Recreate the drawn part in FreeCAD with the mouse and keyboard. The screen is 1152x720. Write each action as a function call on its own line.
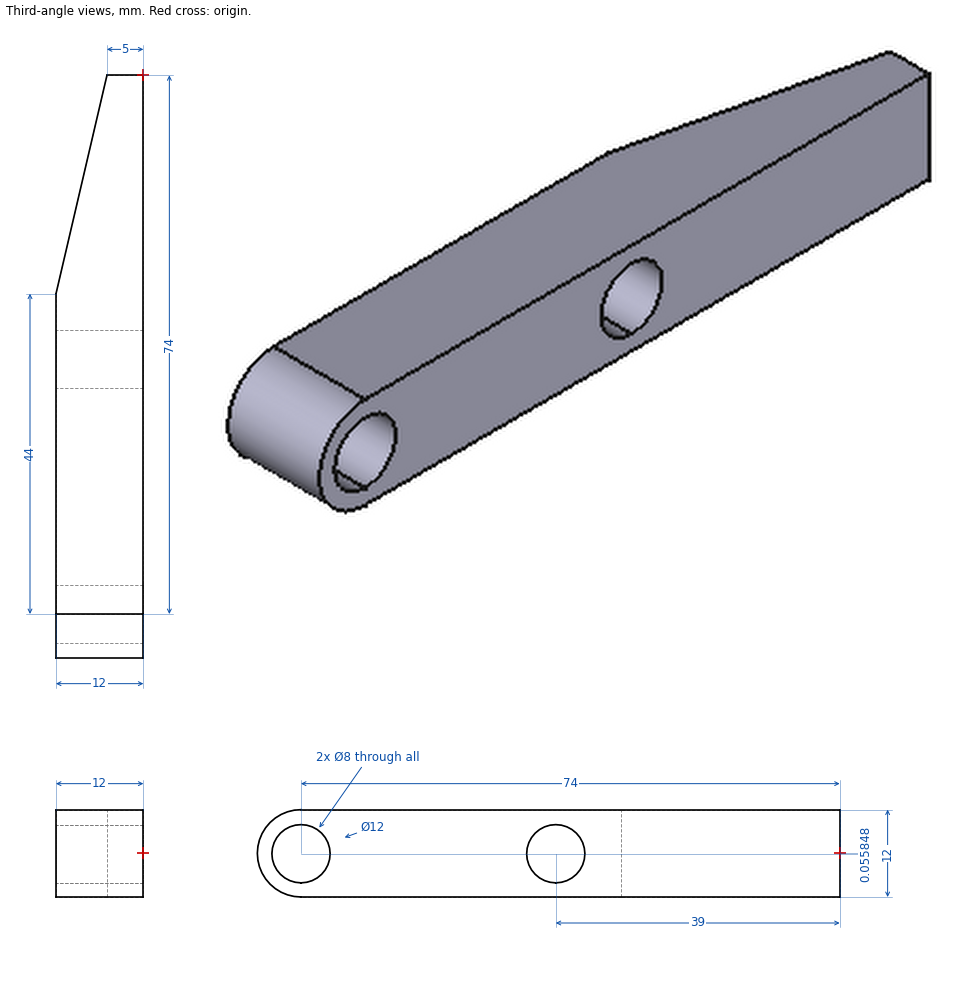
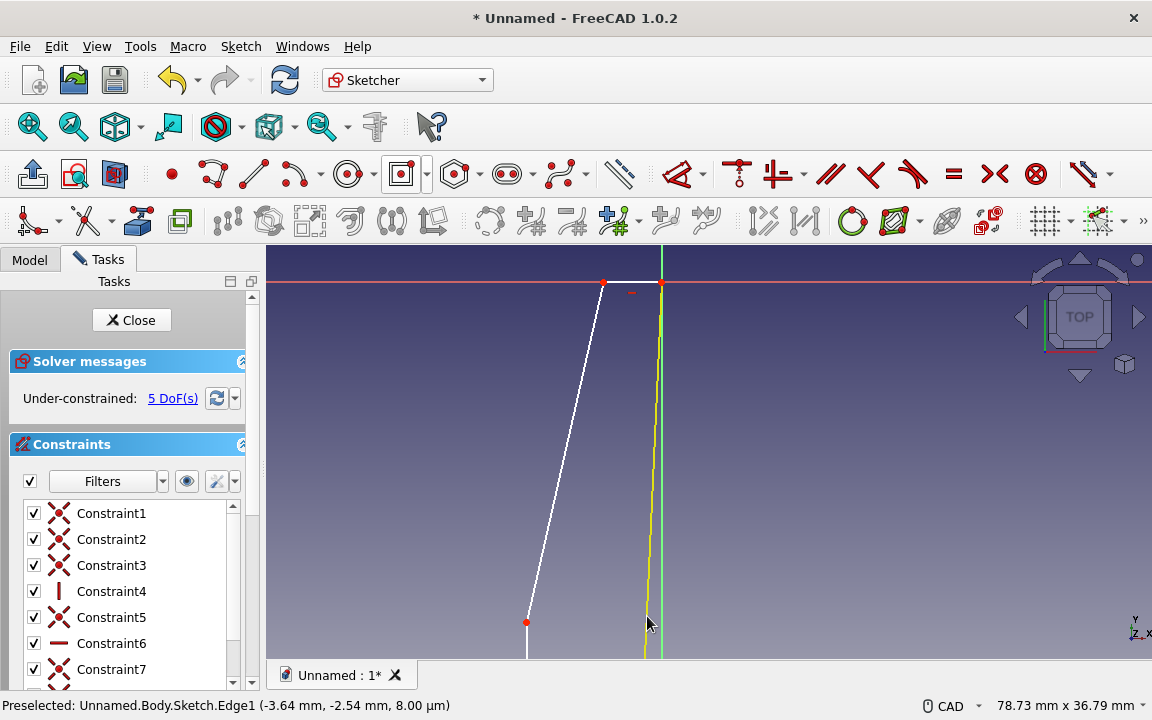
click(647, 616)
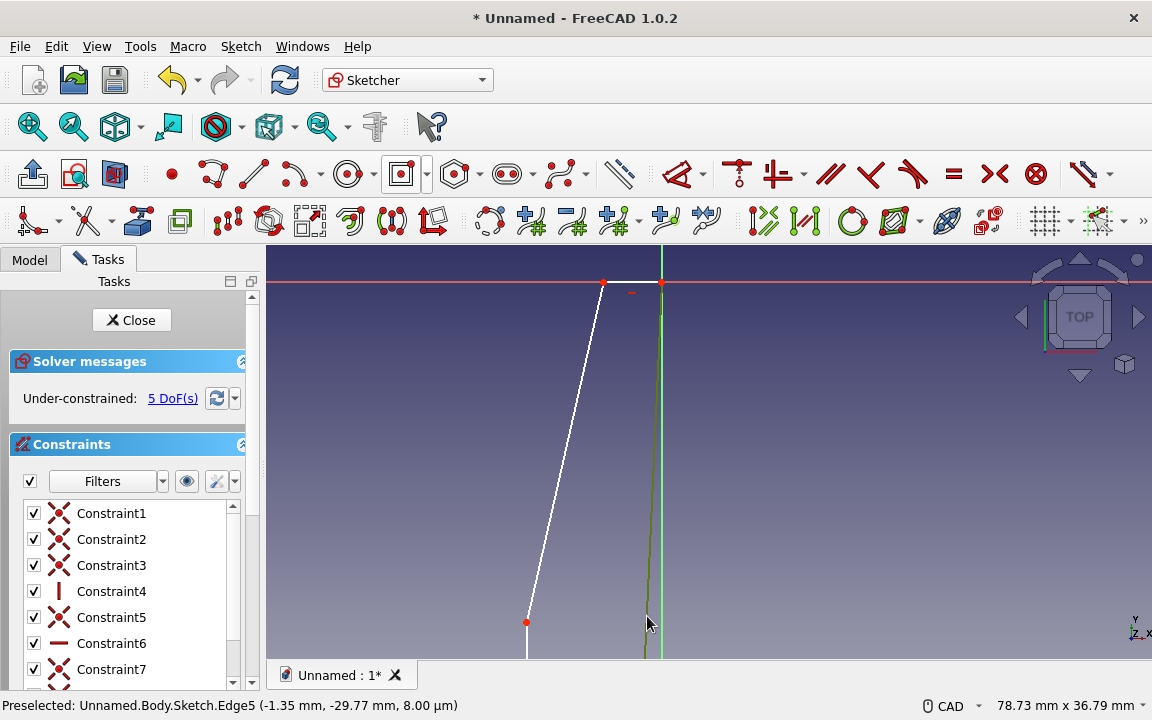
key(v)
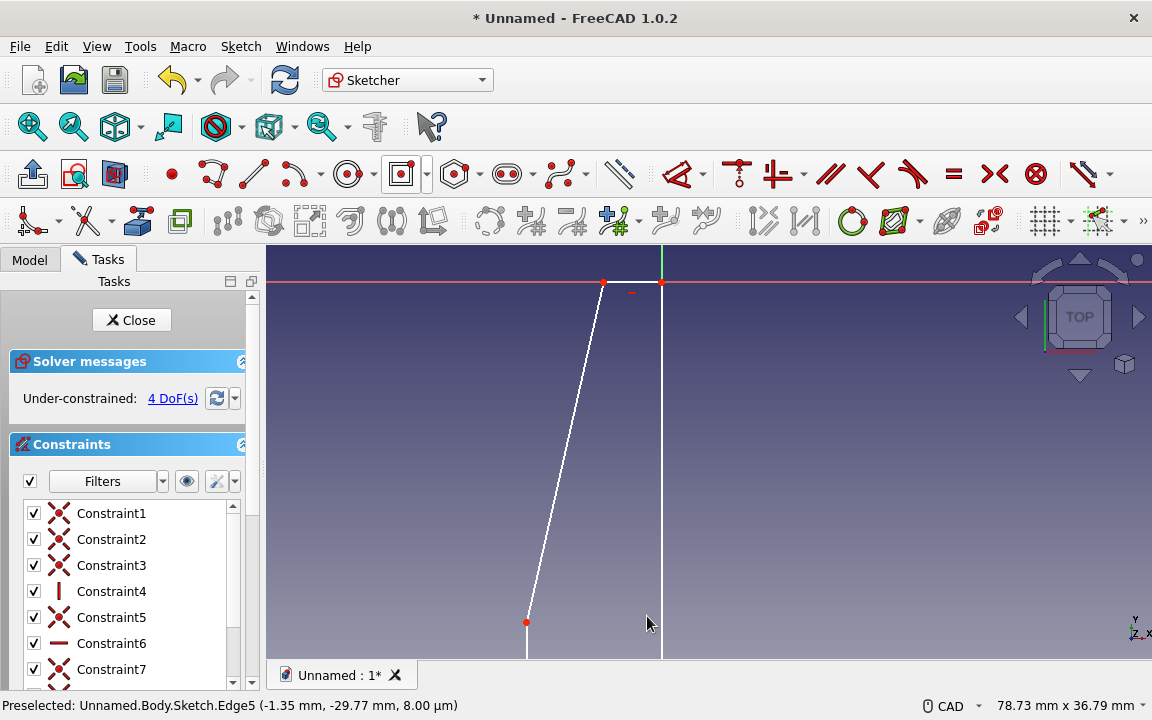
click(645, 282)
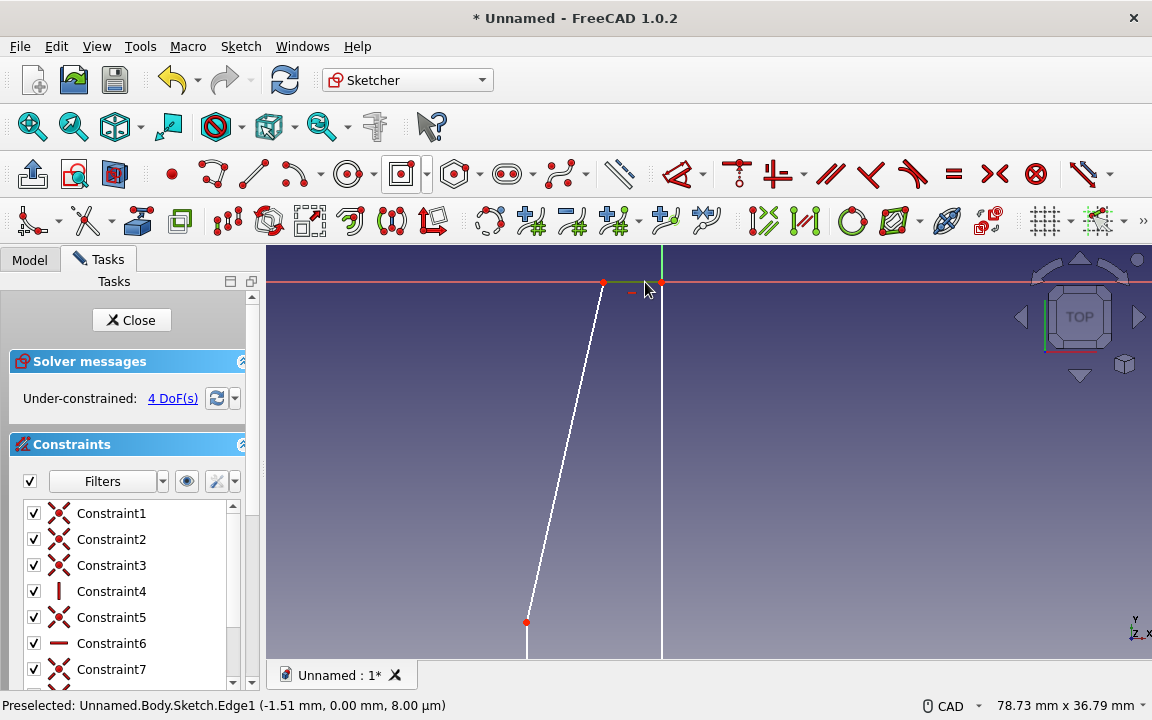
key(l)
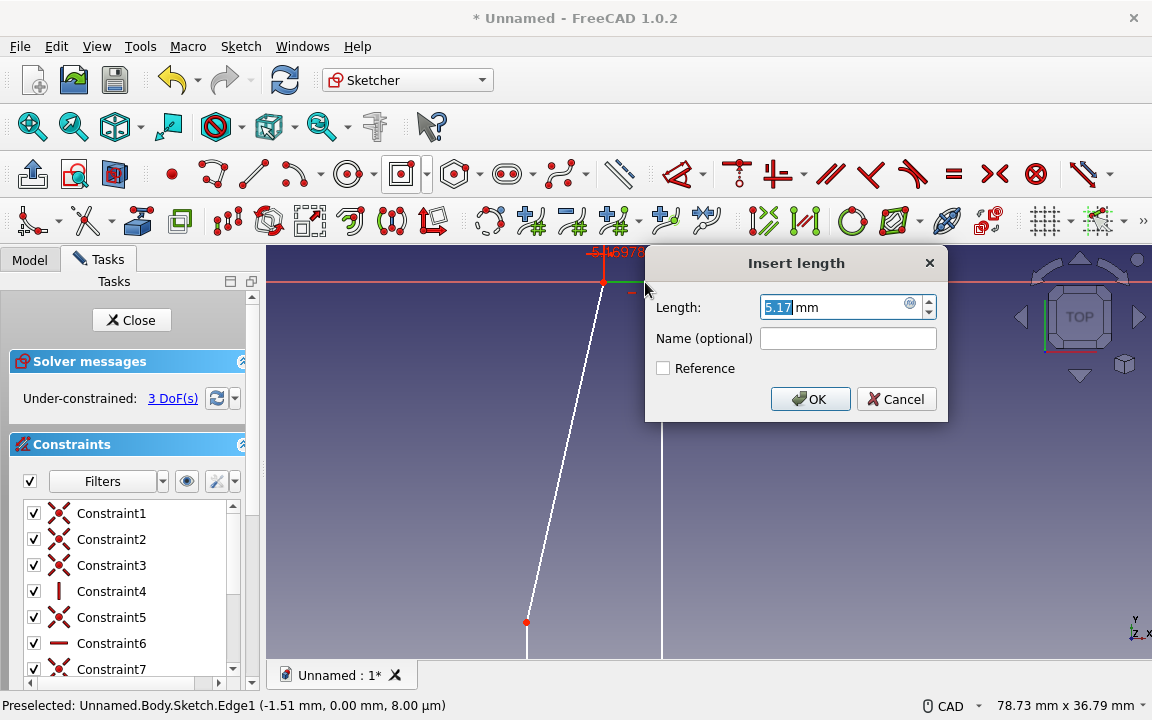
text(5)
key(Return)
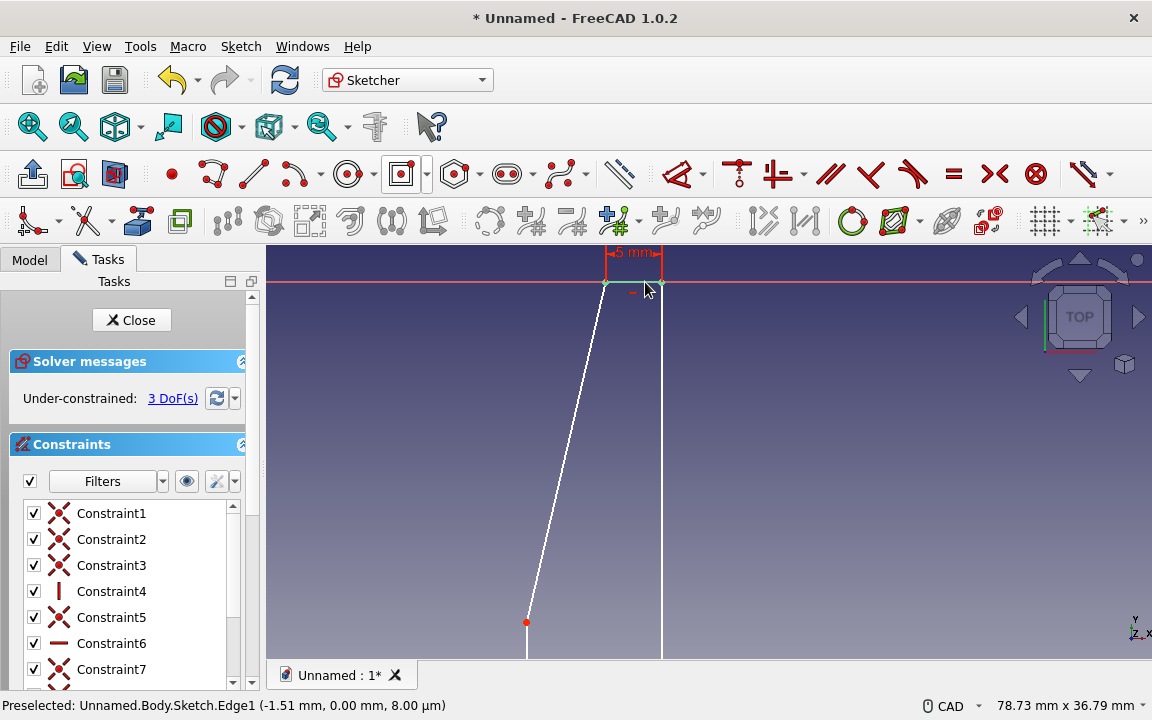
scroll(660, 346, down, 6)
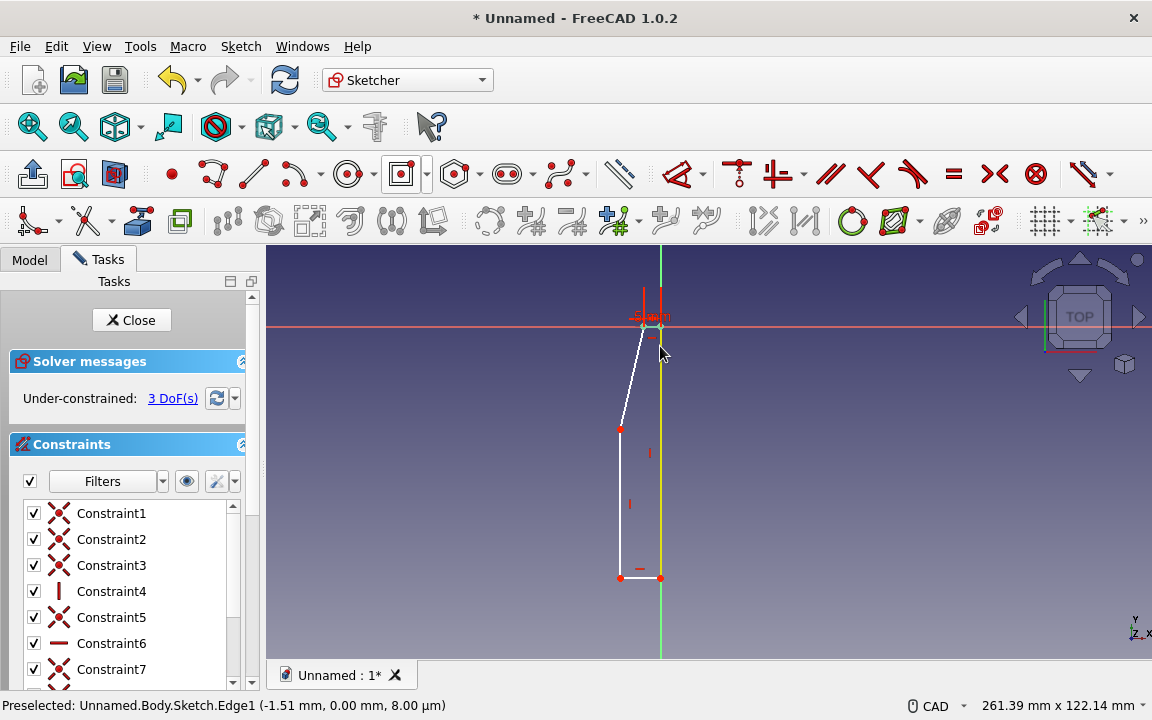
click(620, 474)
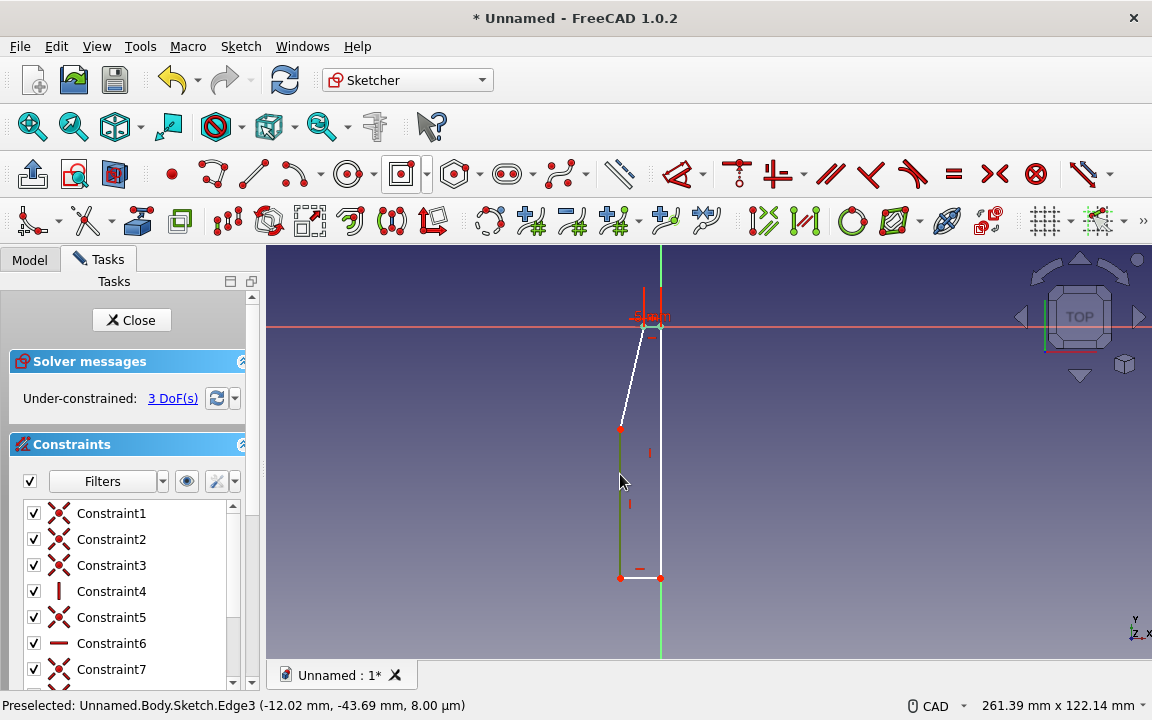
key(i)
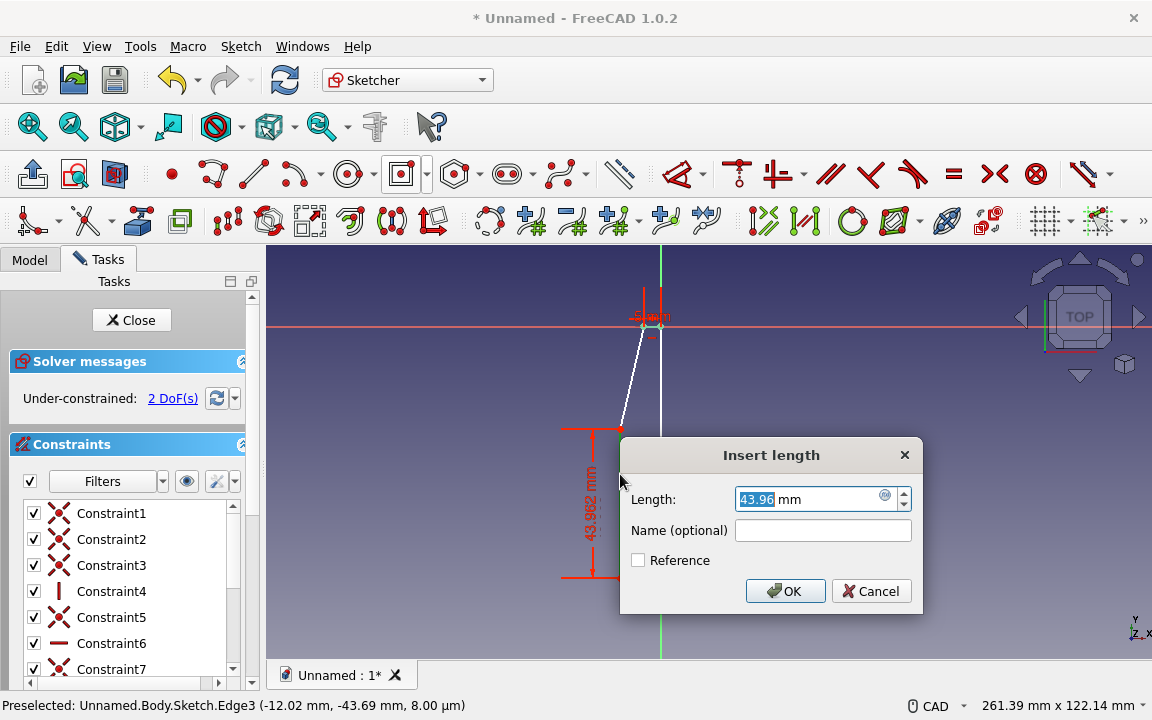
text(44)
key(Return)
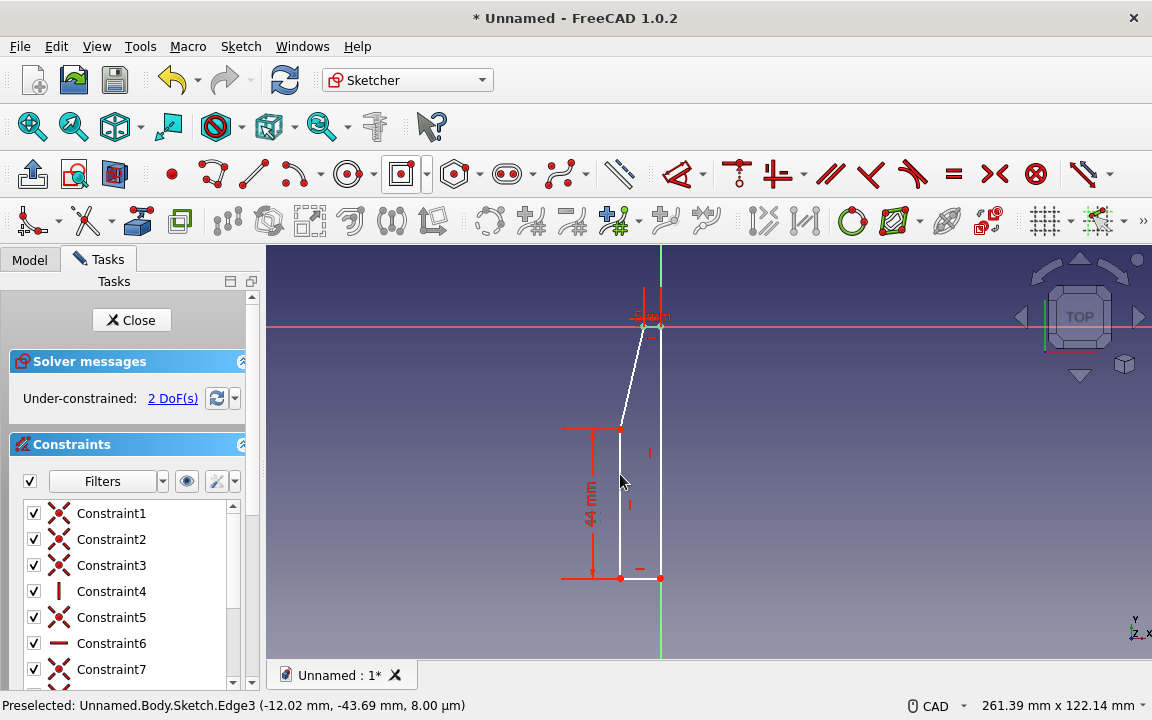
click(632, 579)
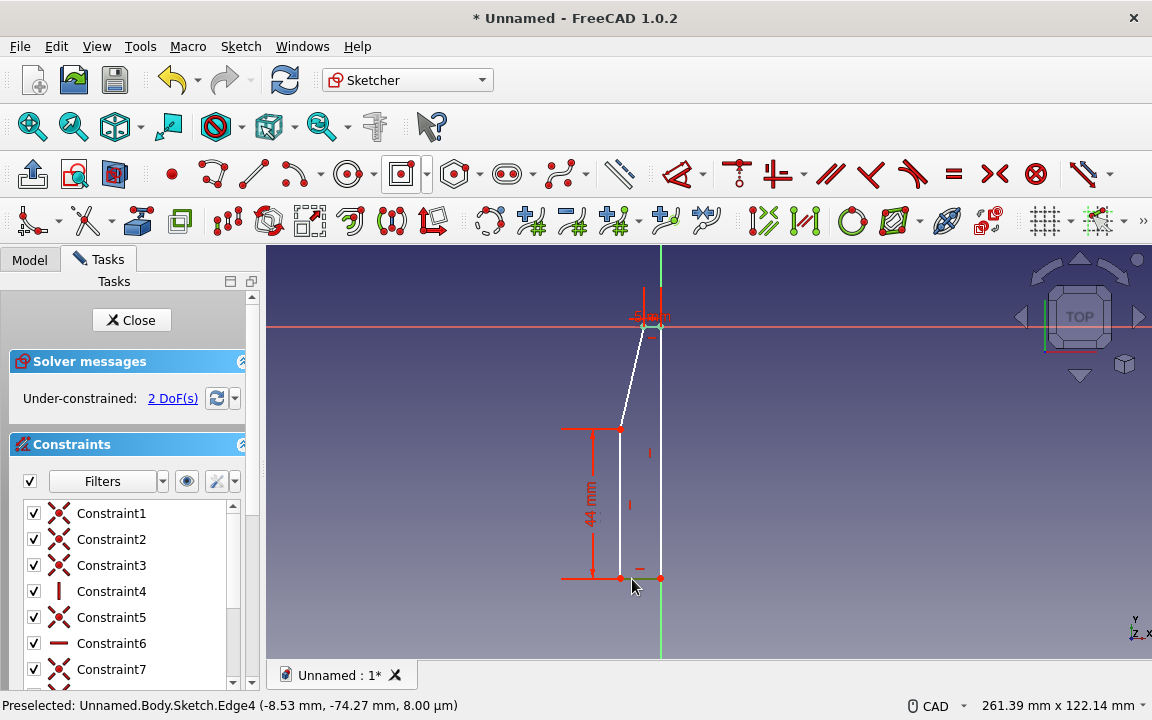
key(l)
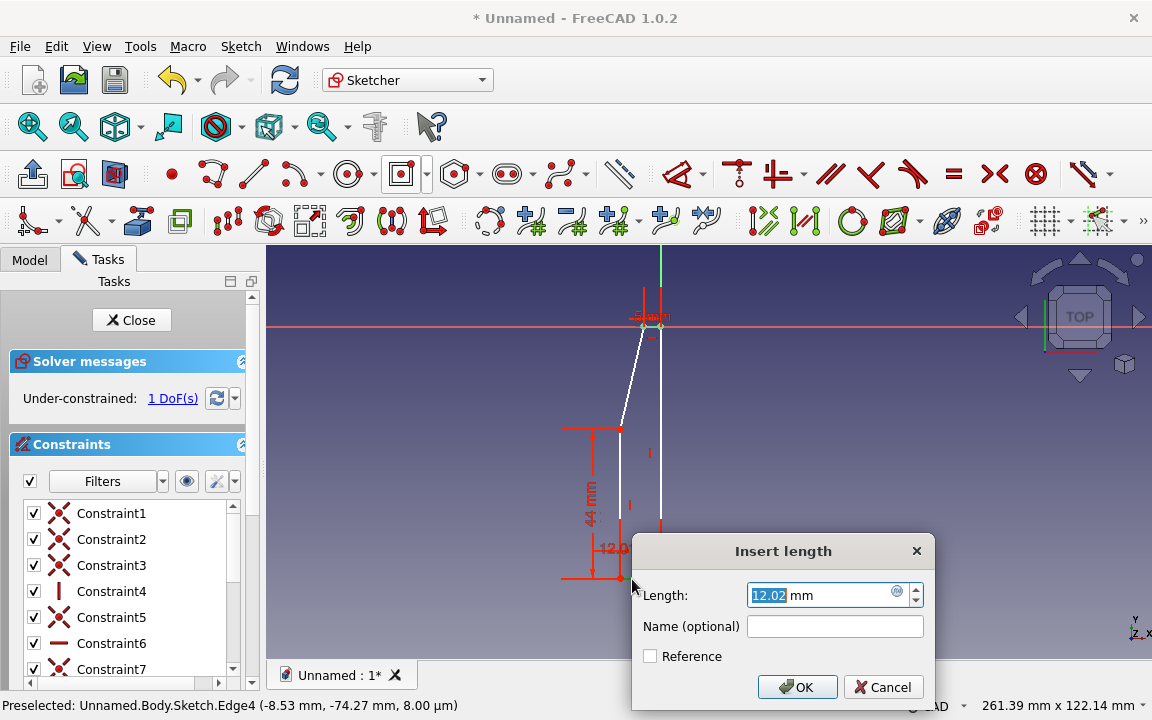
text(12)
key(Return)